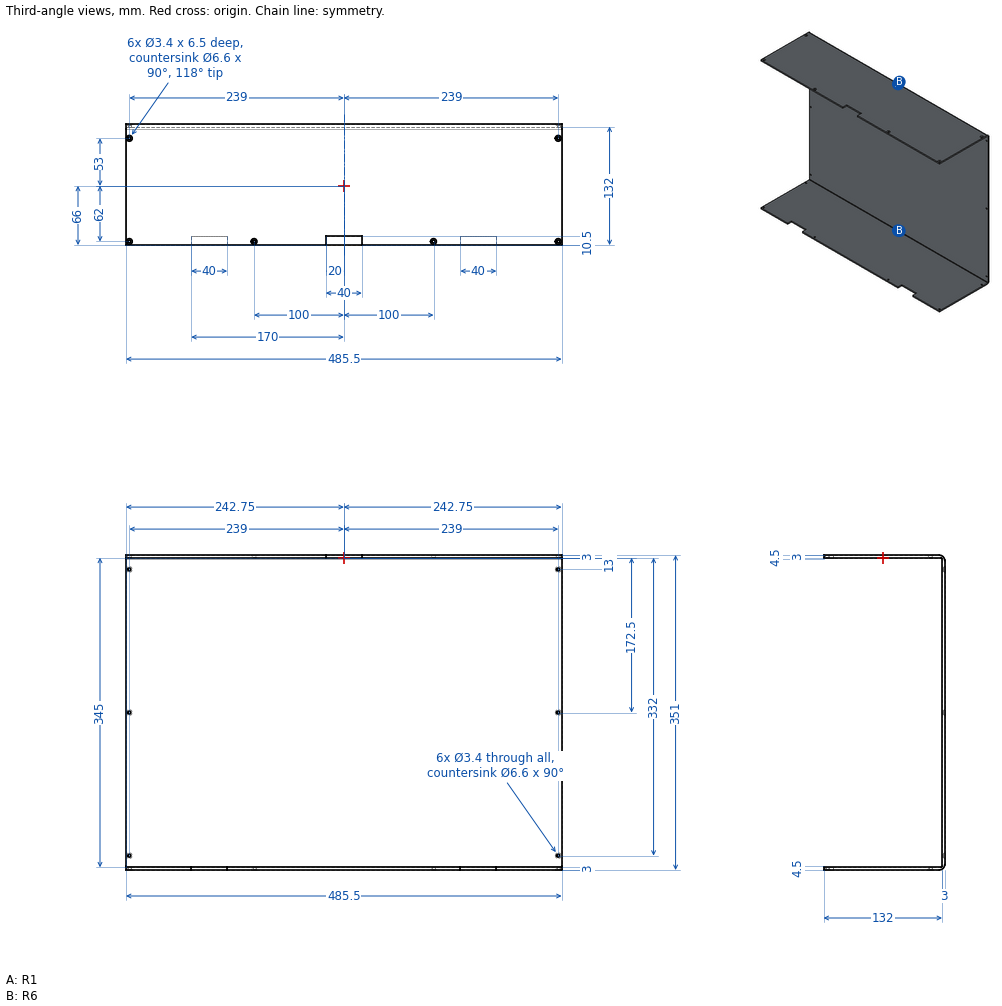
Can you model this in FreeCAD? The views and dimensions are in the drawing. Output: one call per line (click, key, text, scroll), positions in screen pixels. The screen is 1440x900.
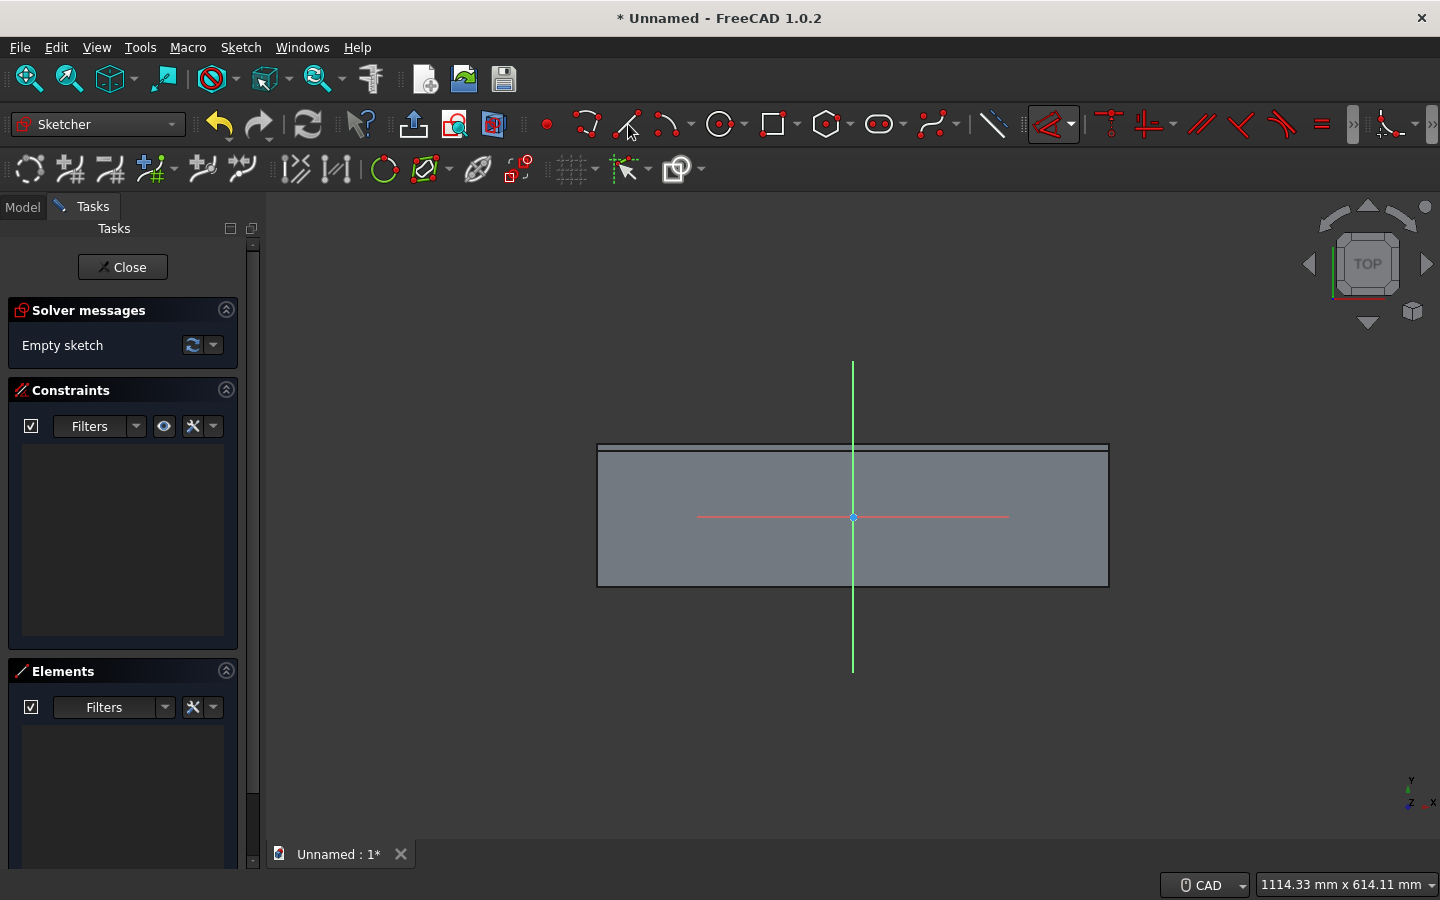
scroll(867, 559, up, 9)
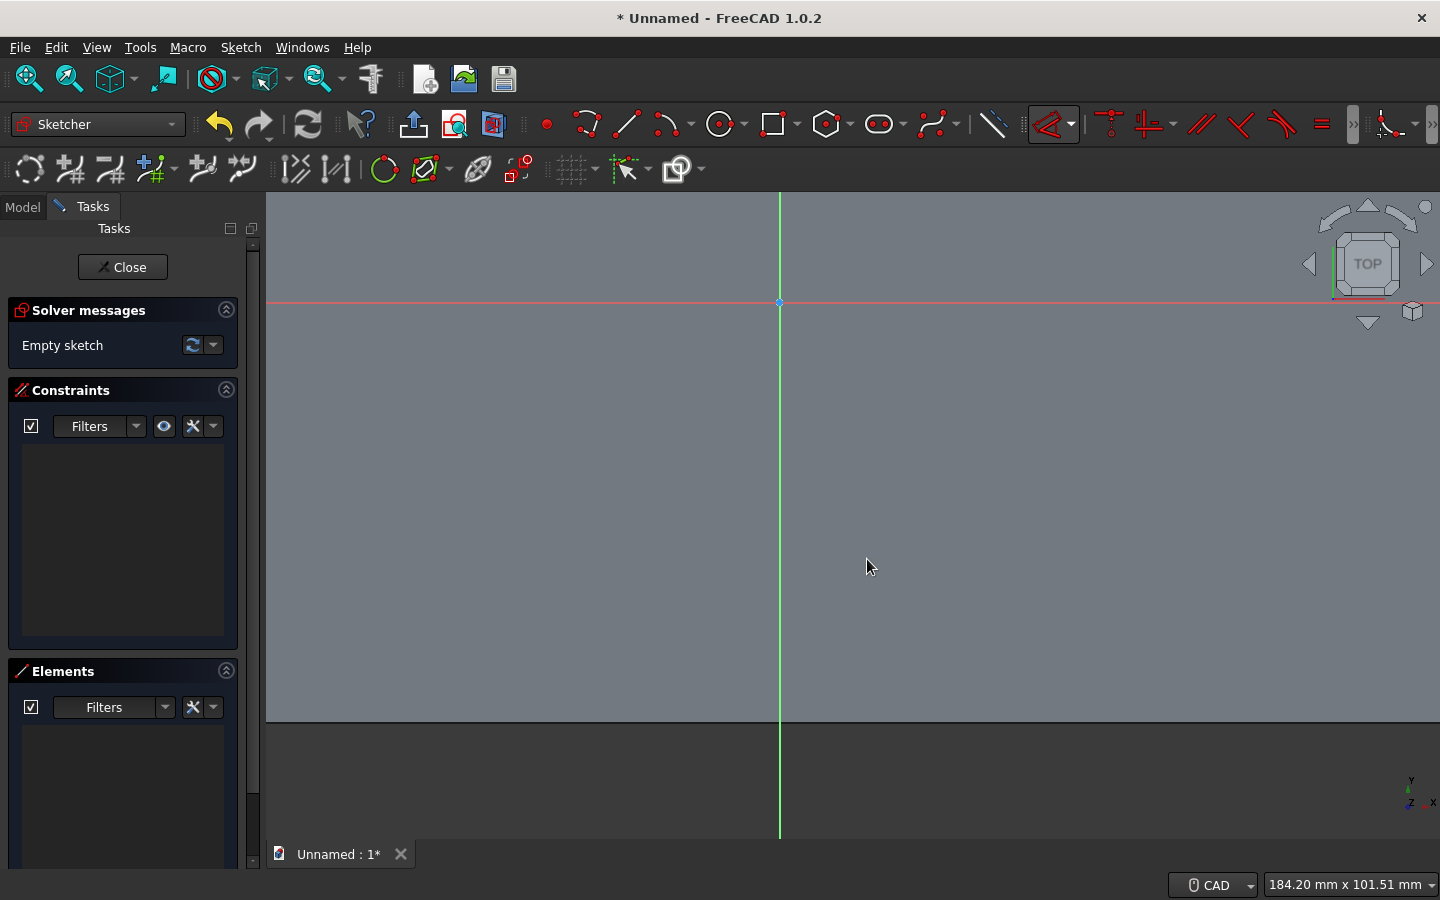
click(774, 124)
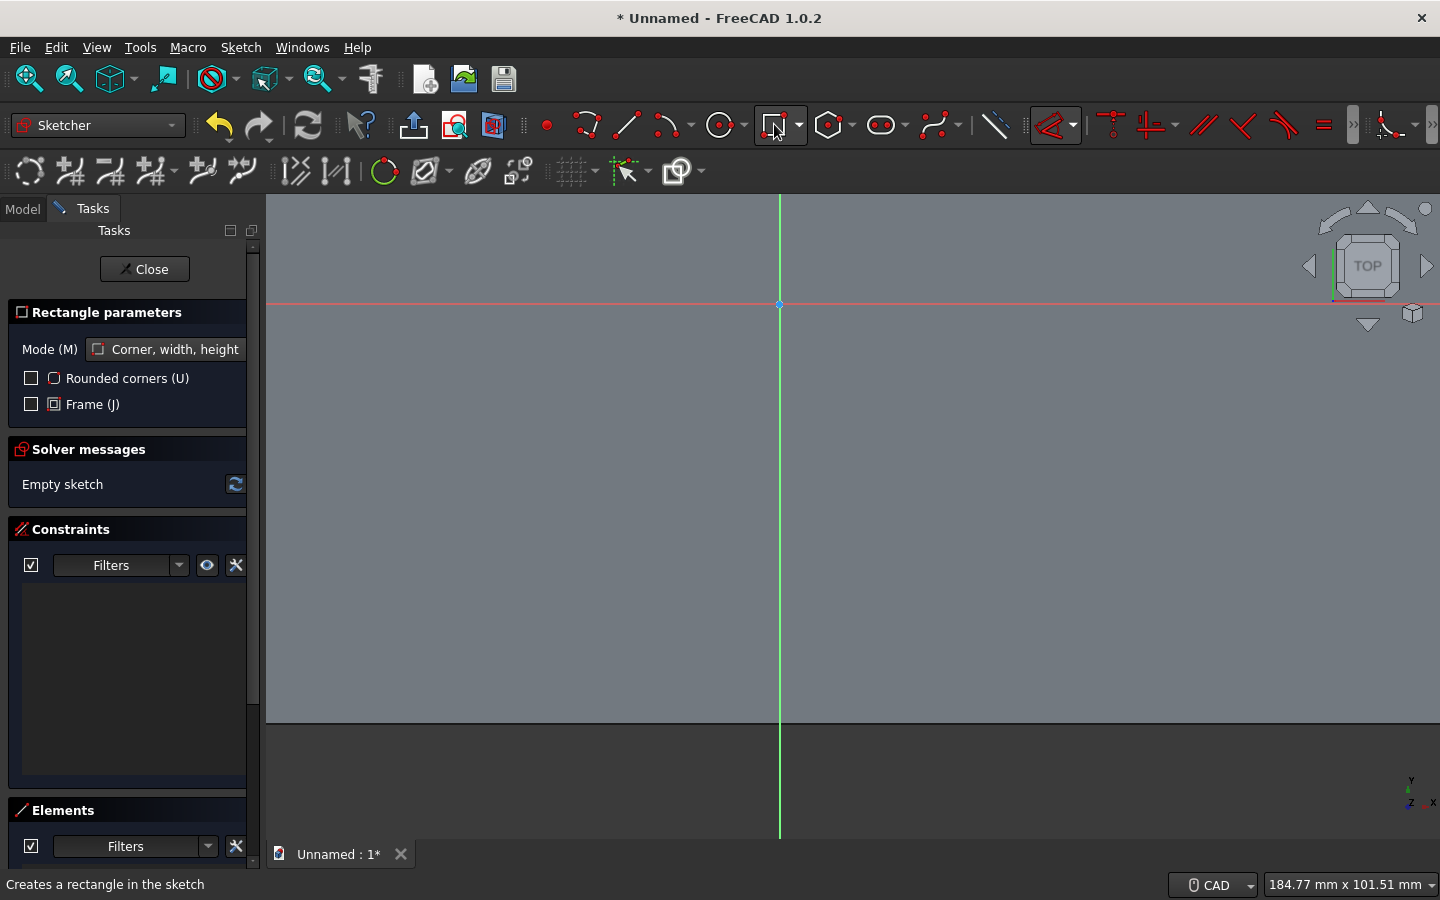
click(653, 657)
move(907, 724)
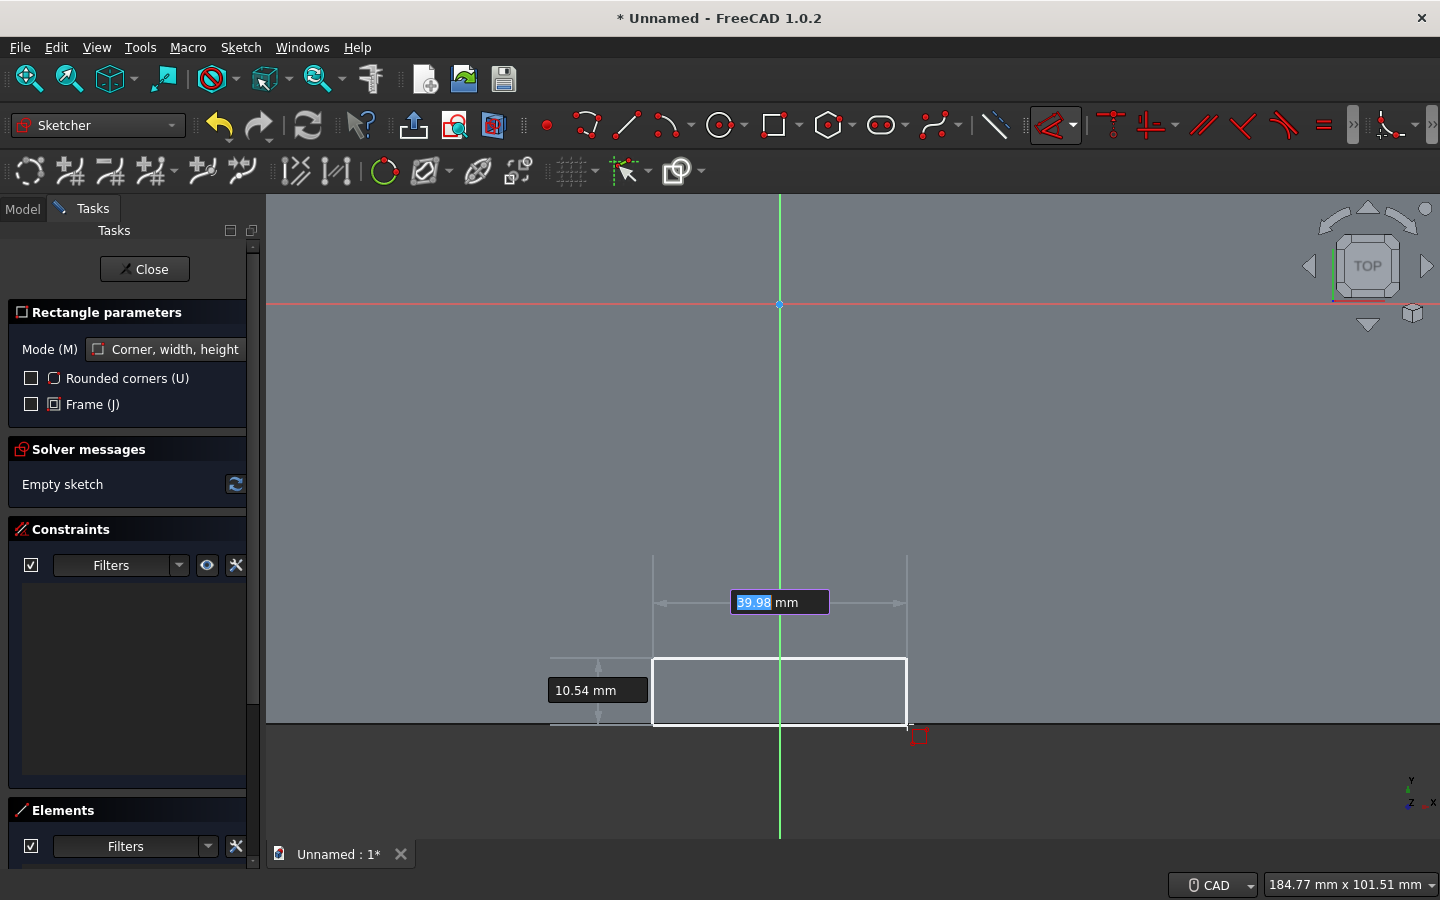
text(40)
key(Tab)
text(10.5)
key(Return)
key(Escape)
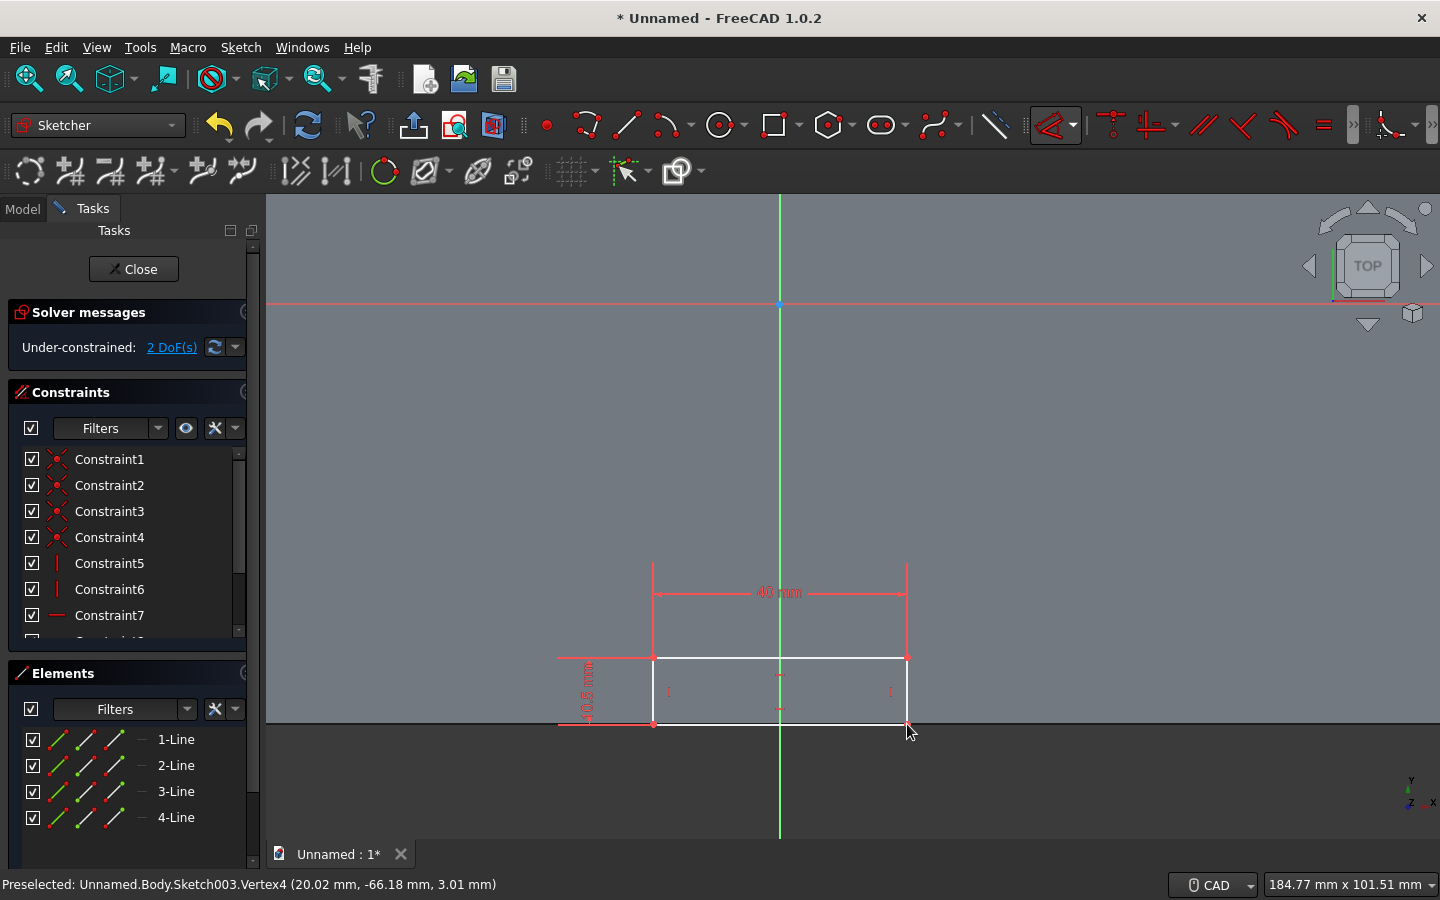
click(653, 658)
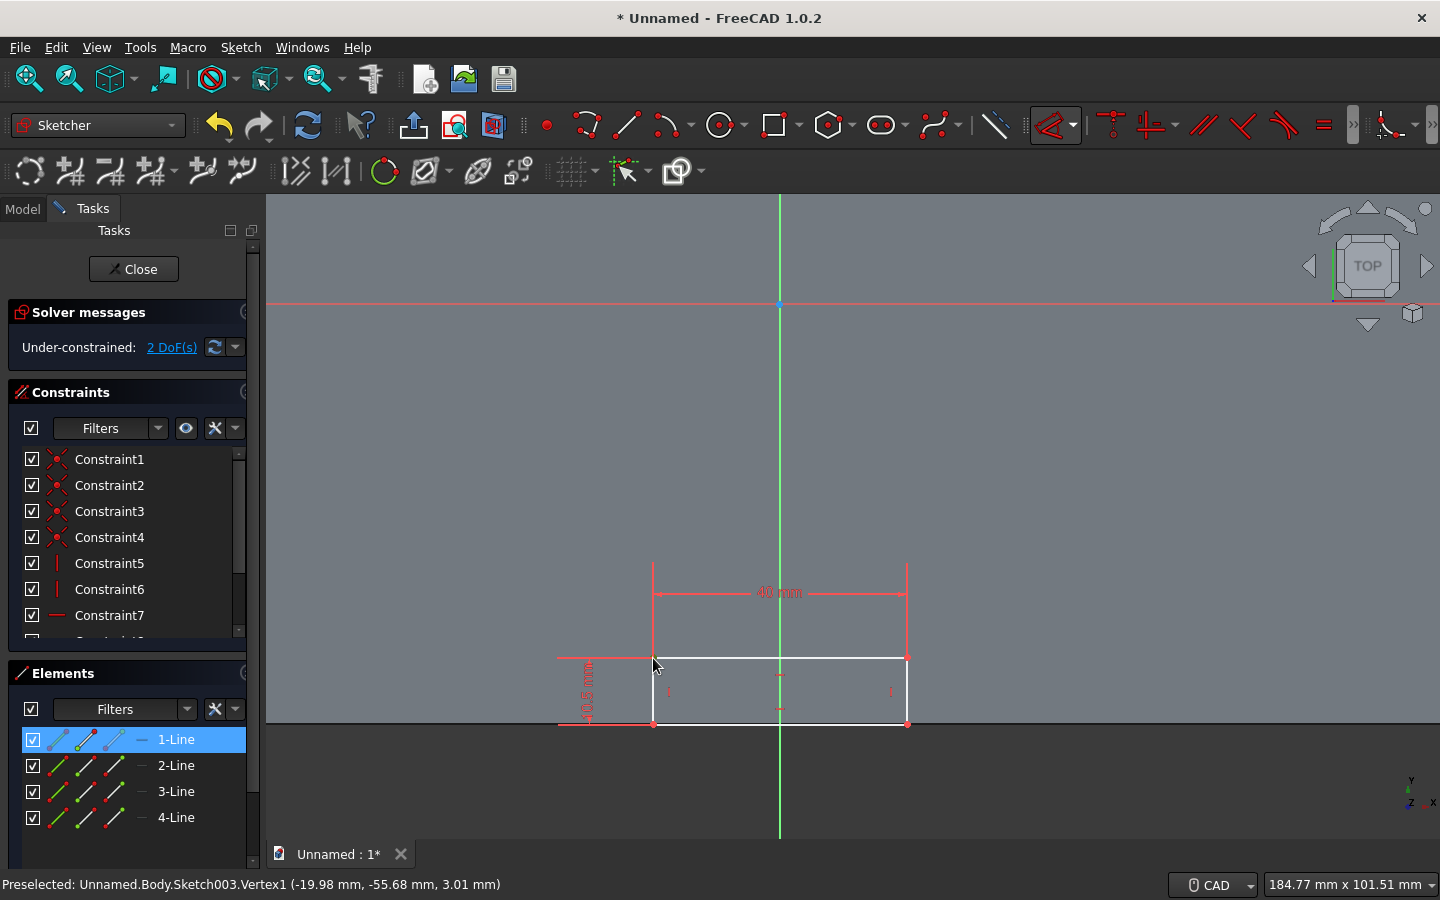
key(l)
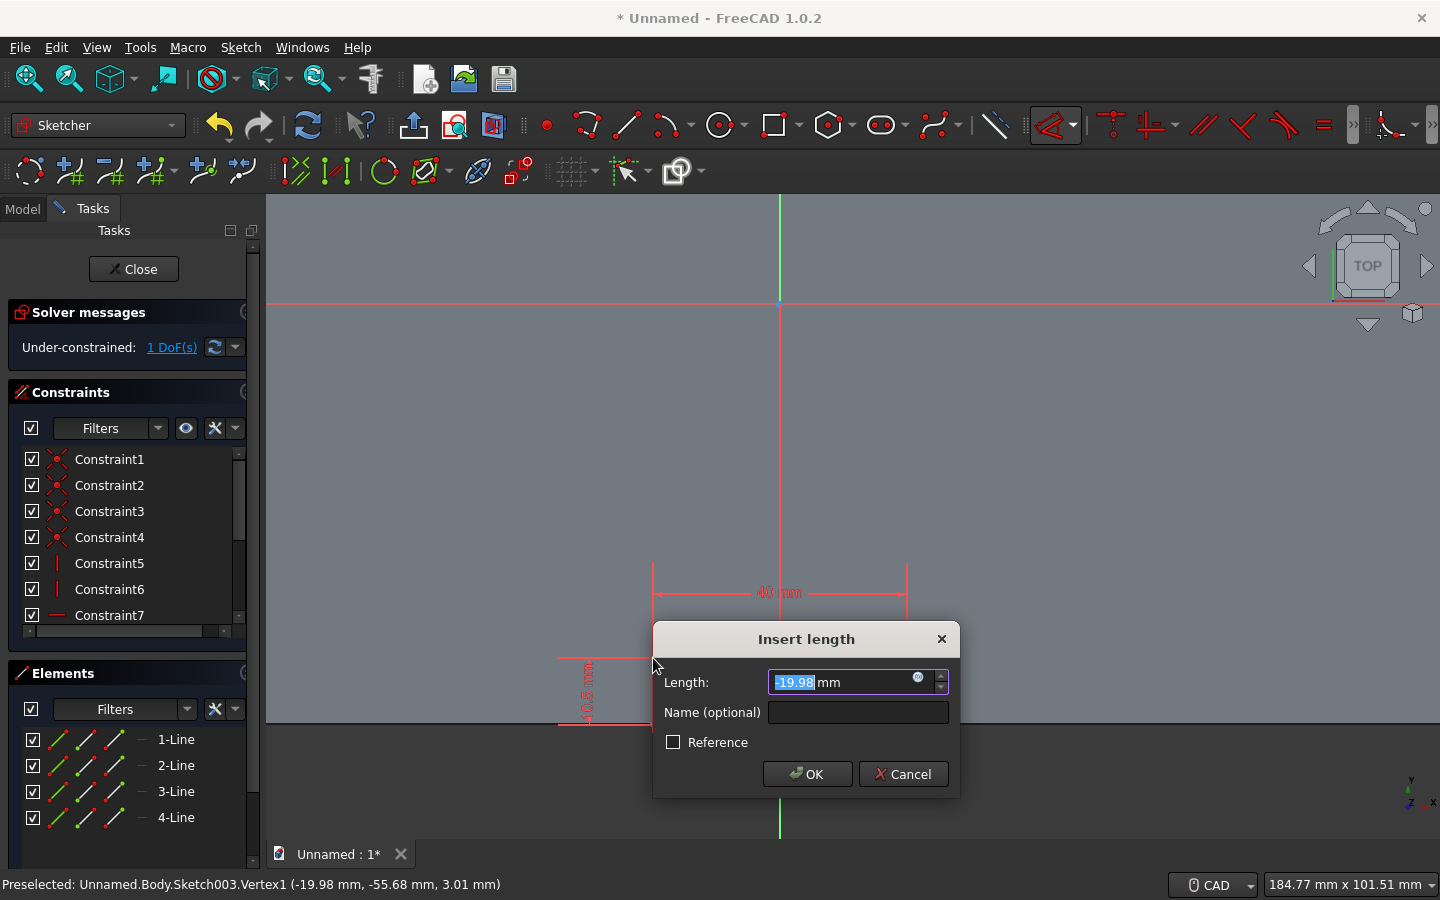
text(-20)
key(Return)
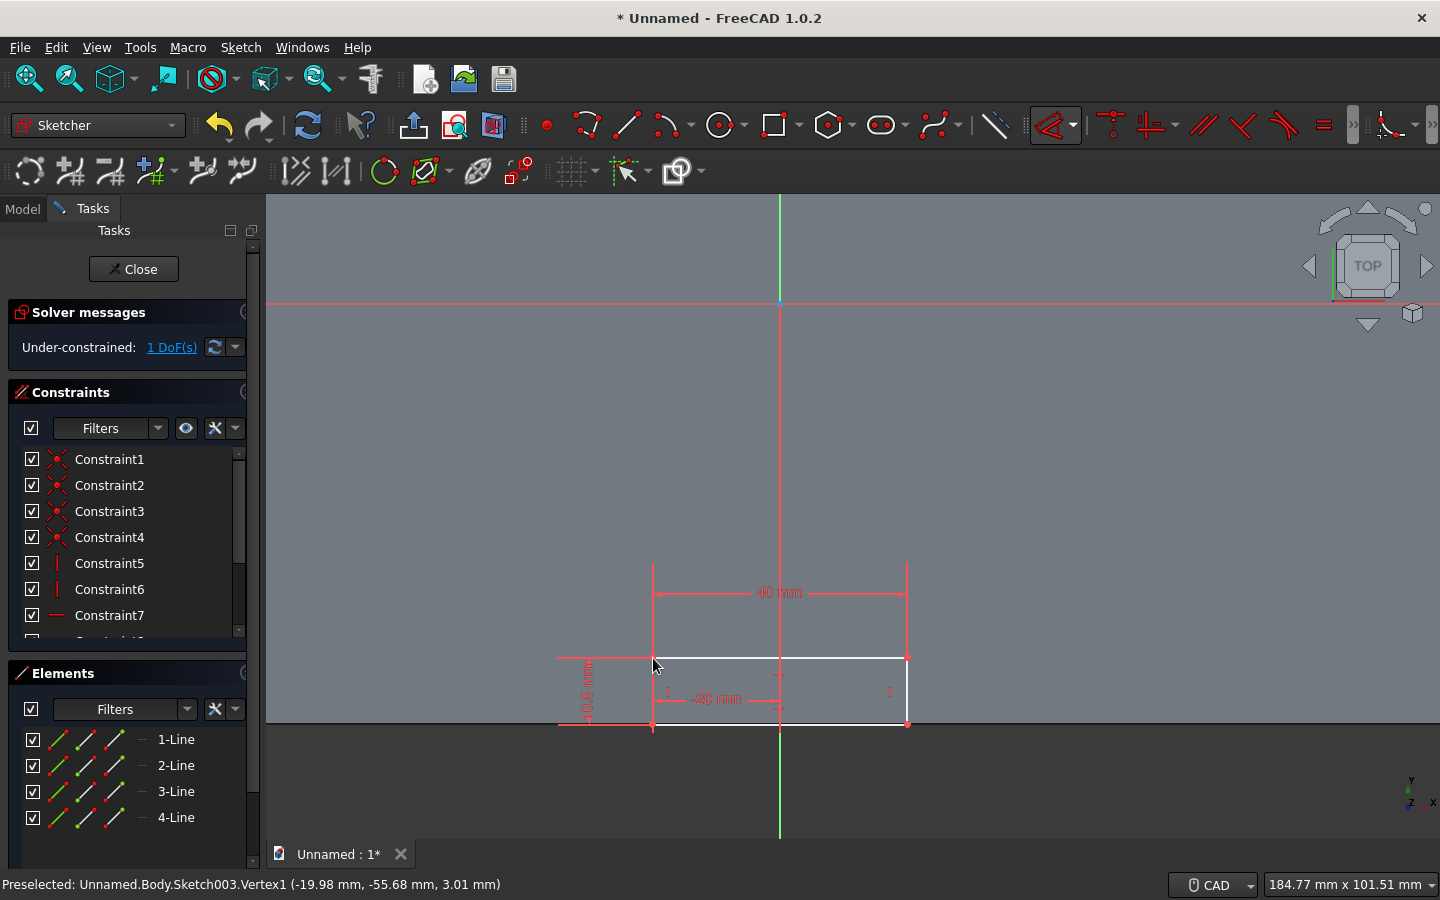
click(653, 725)